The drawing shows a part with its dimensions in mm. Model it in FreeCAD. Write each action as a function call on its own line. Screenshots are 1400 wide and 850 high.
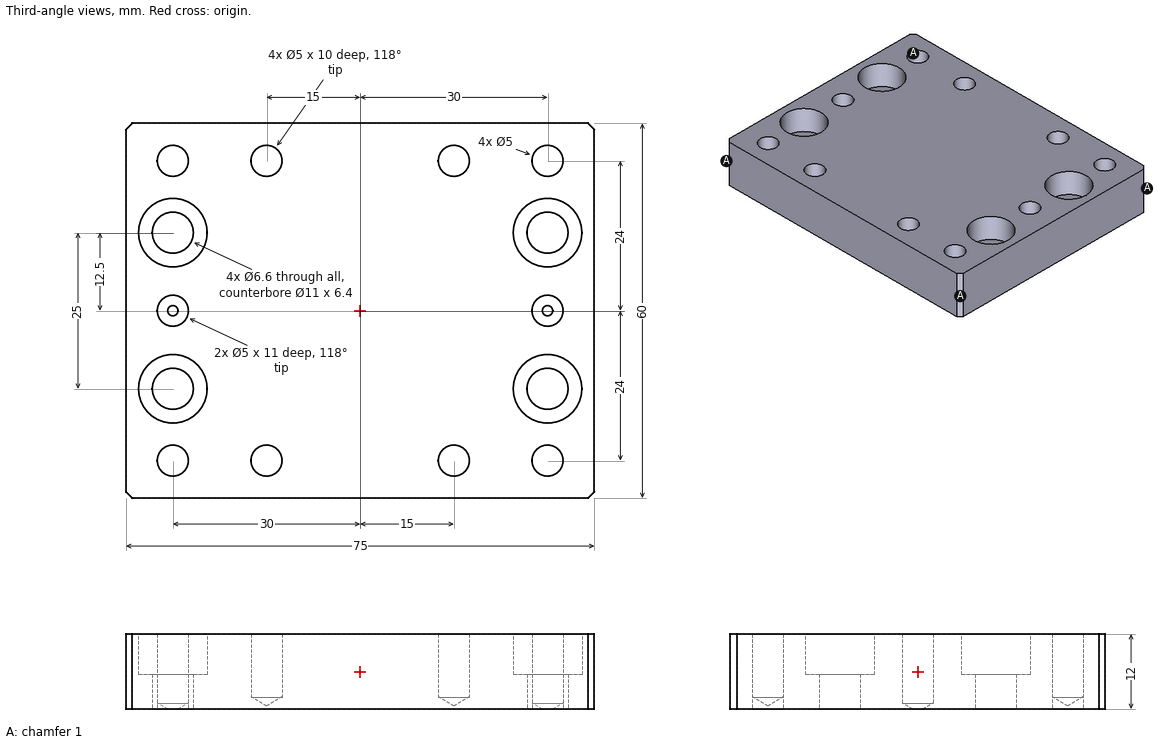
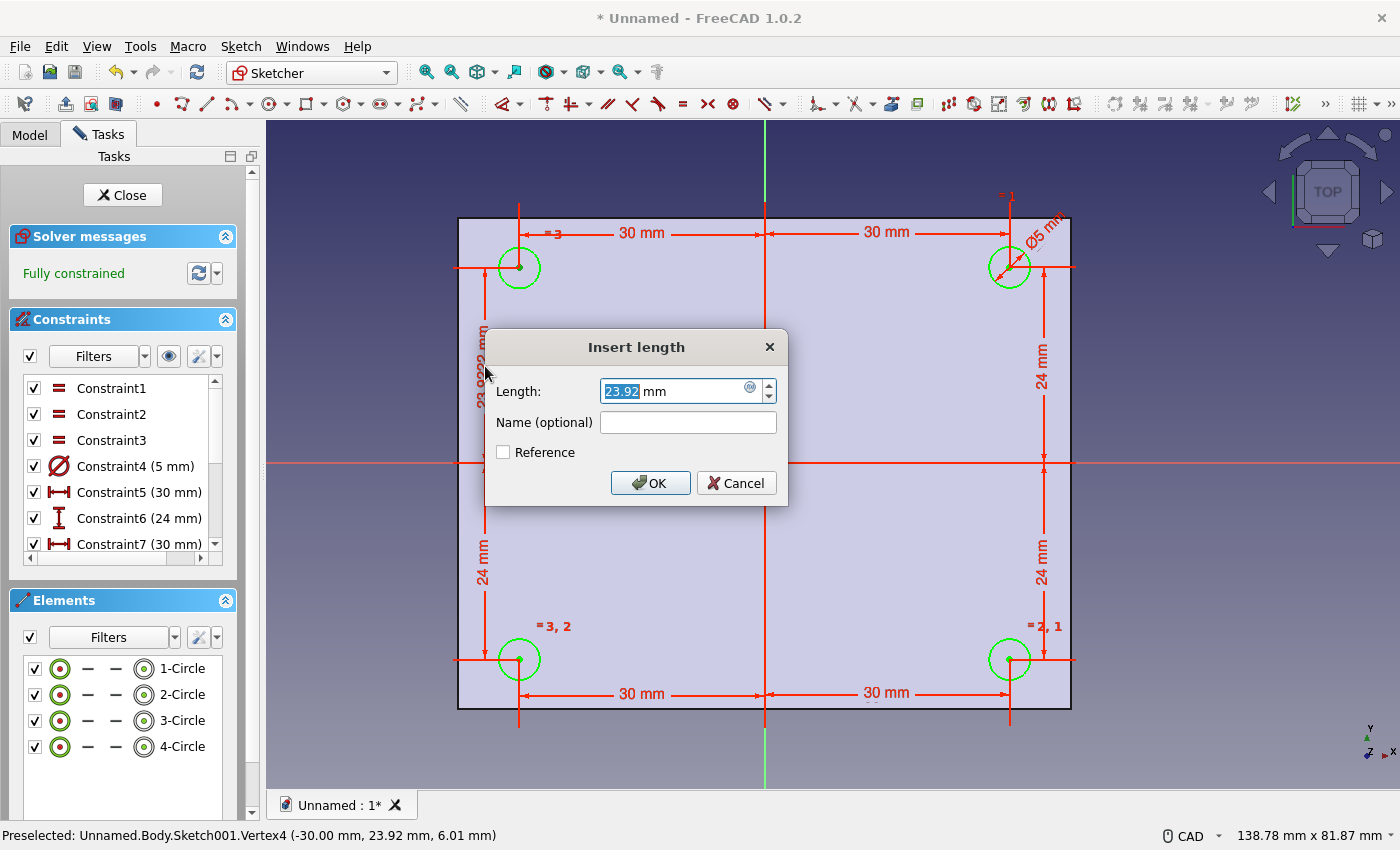
text(24)
key(Return)
key(Escape)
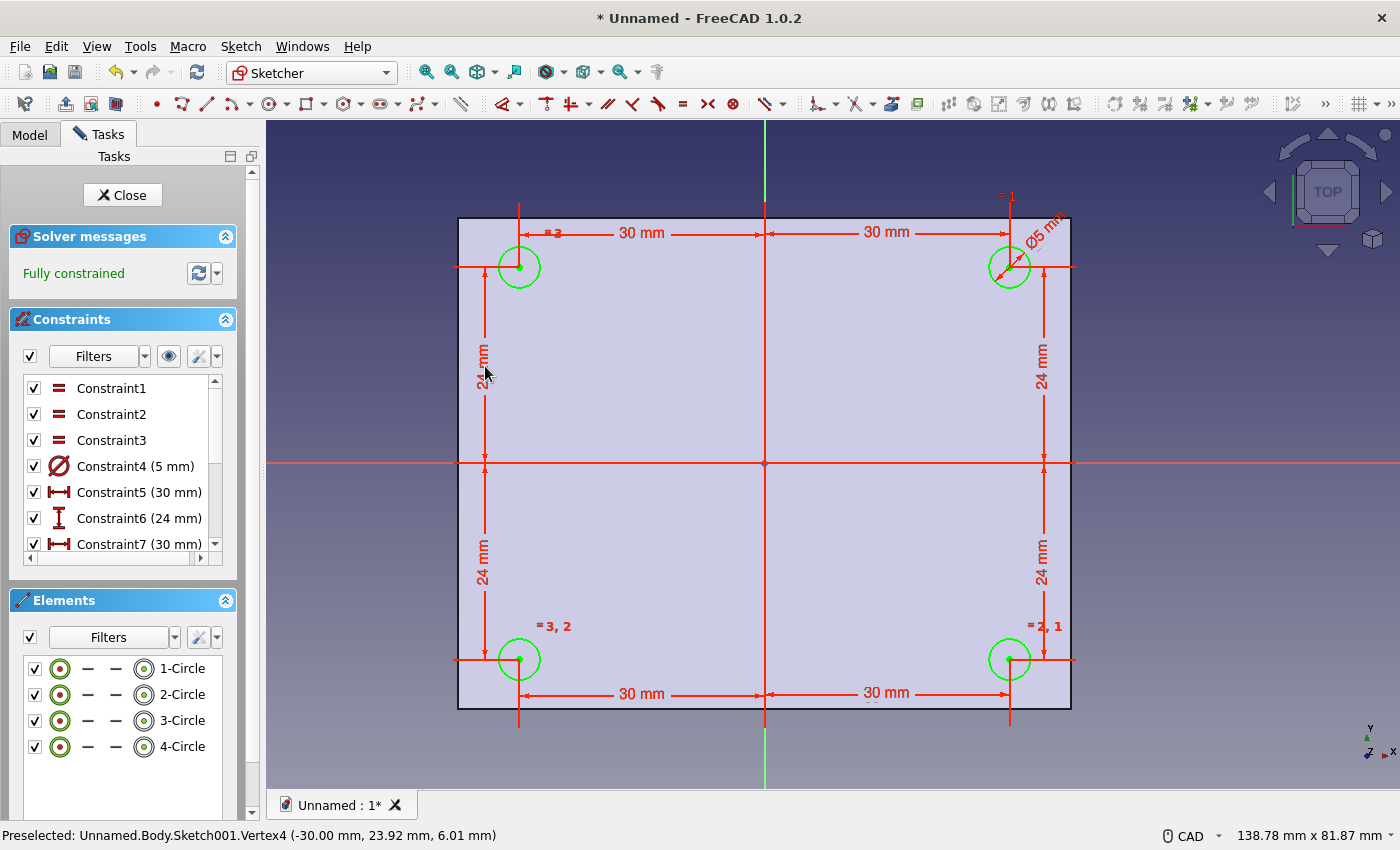
click(123, 195)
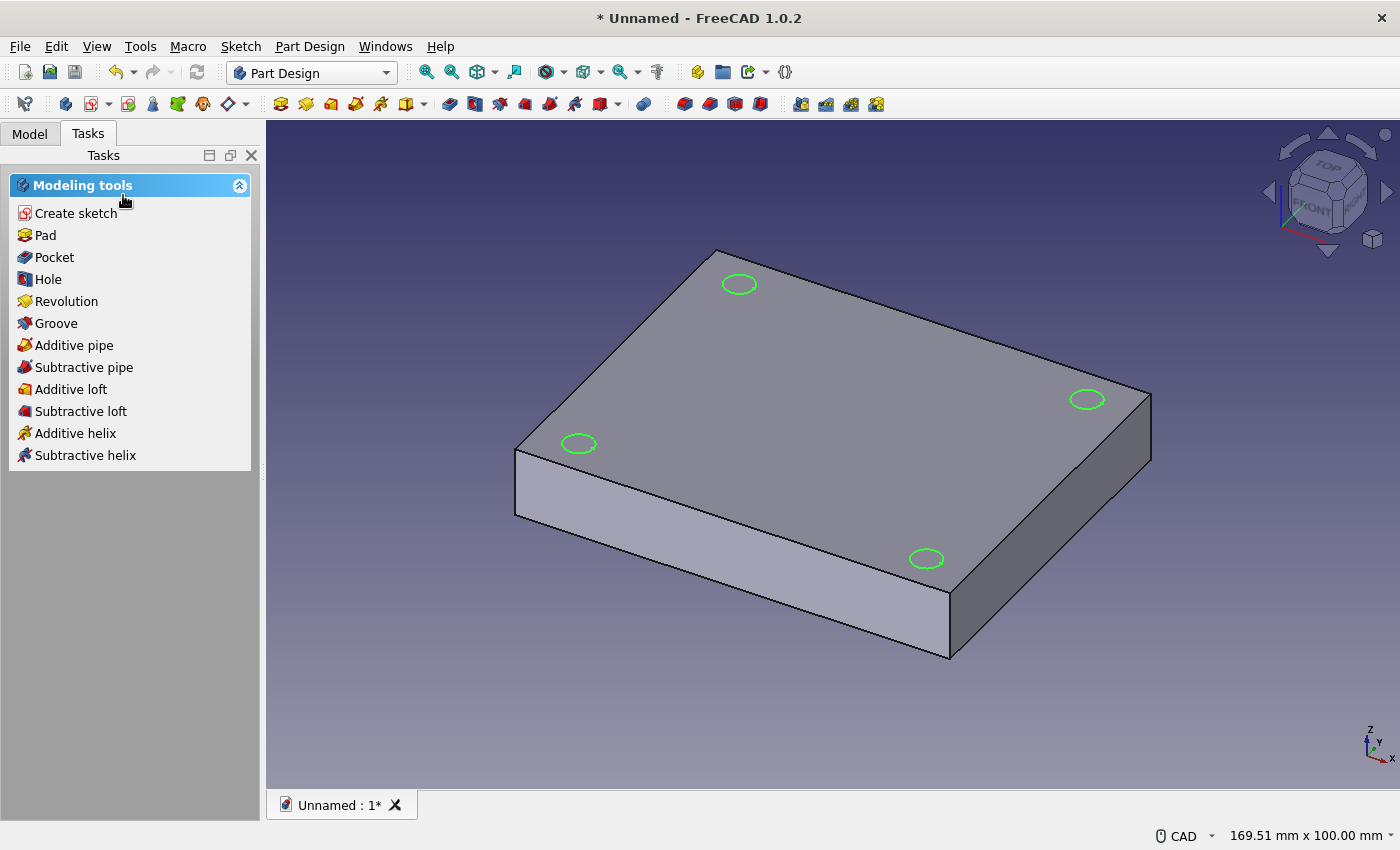
click(450, 104)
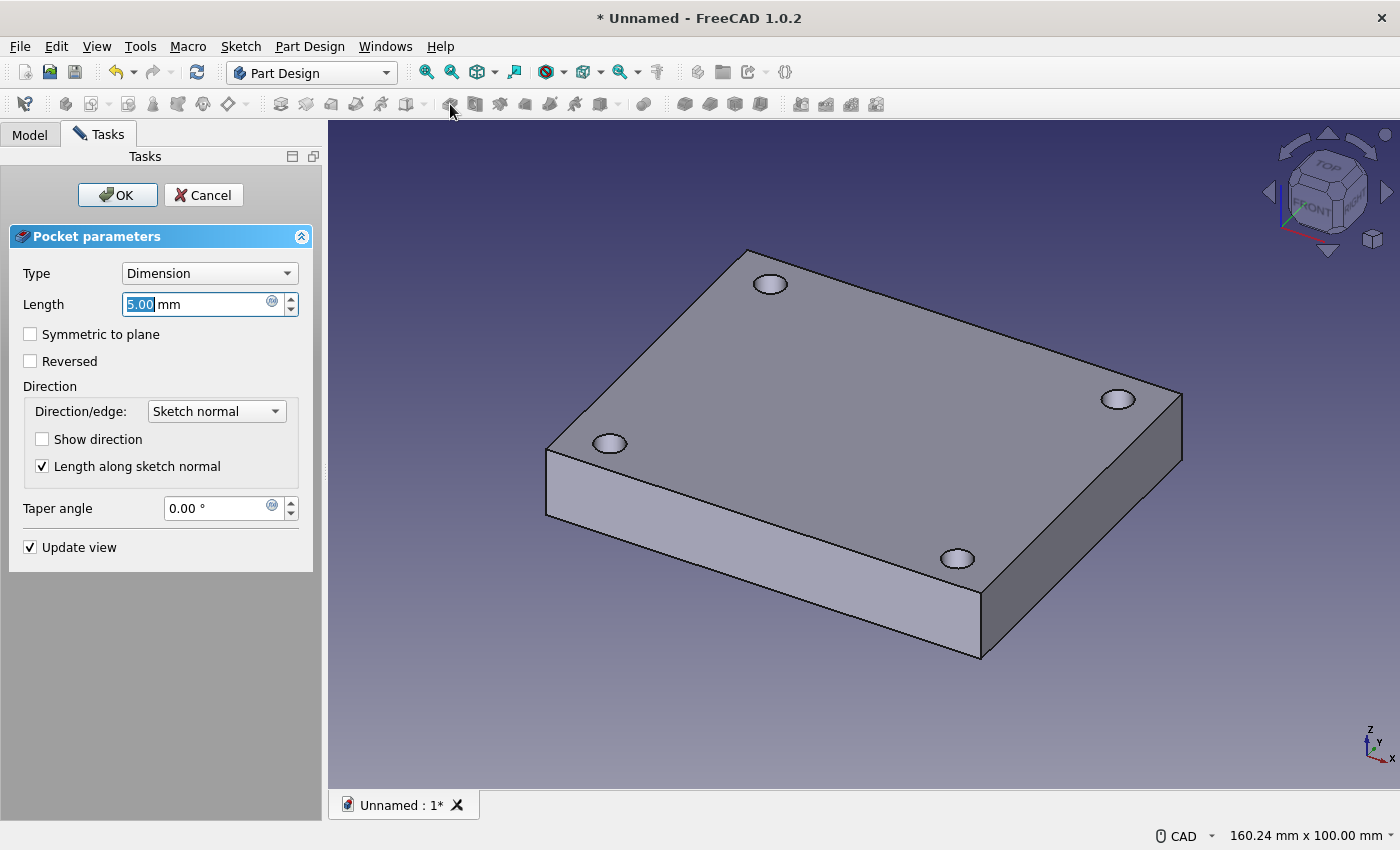
click(210, 274)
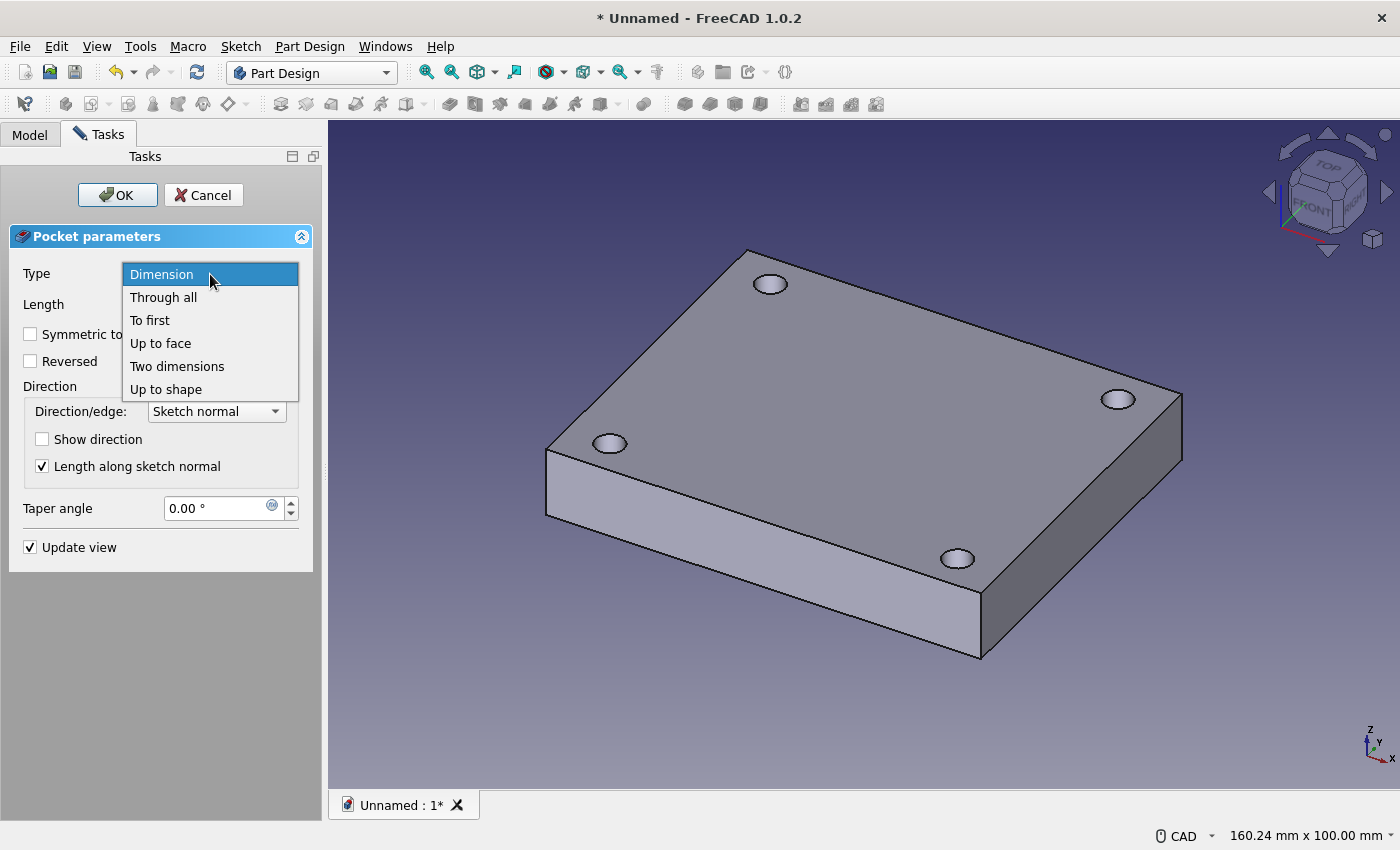
click(208, 298)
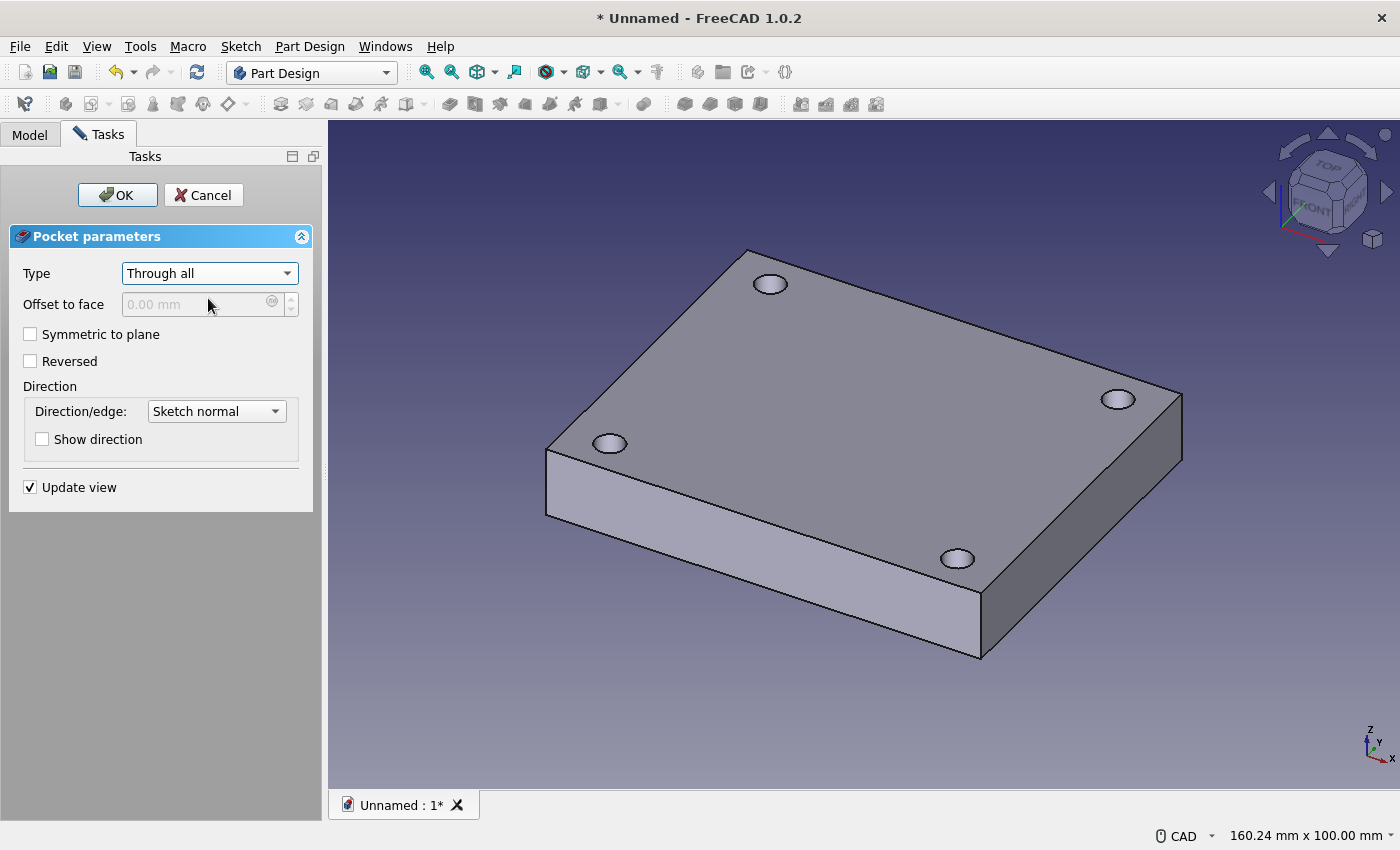
click(118, 195)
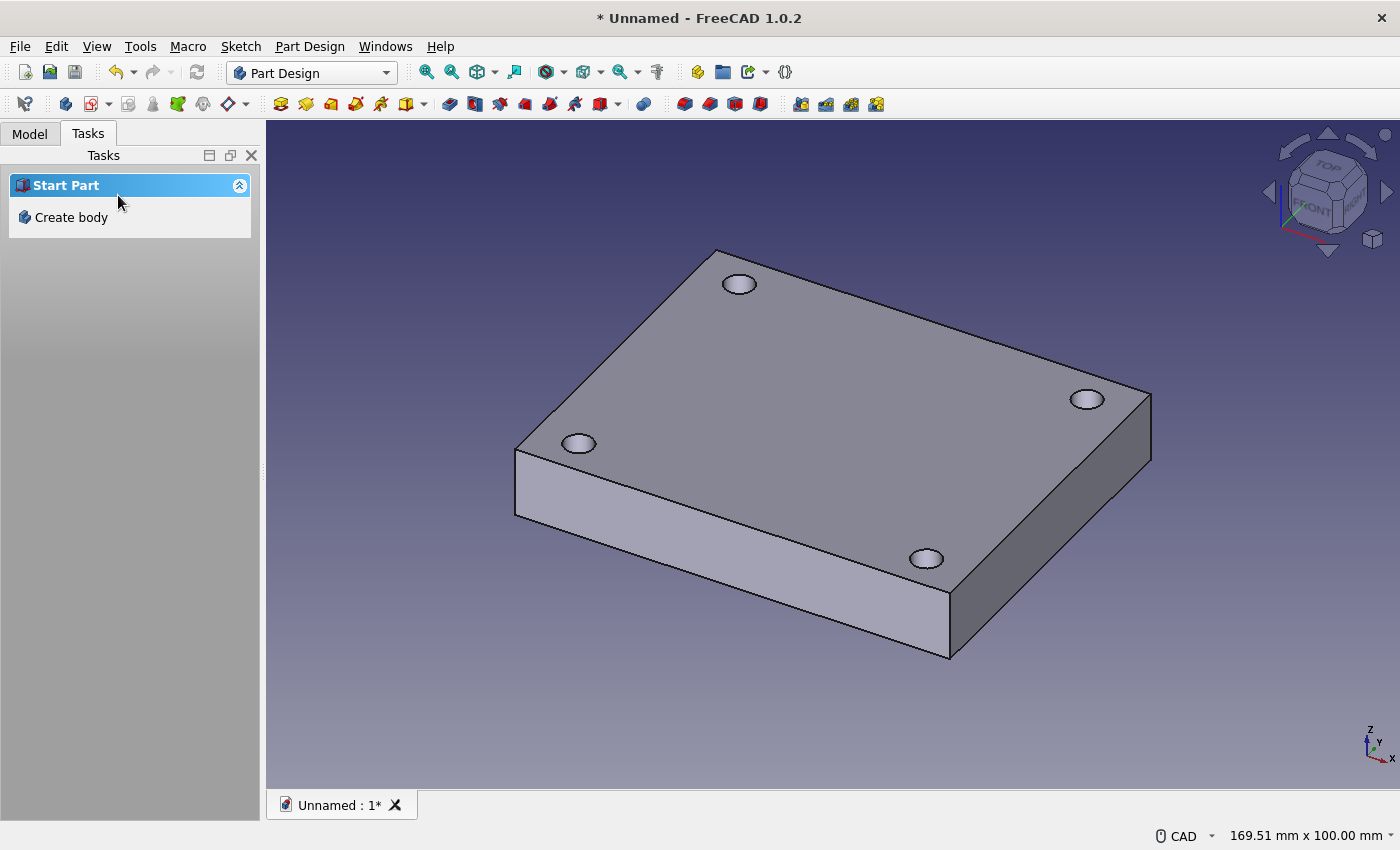
click(833, 421)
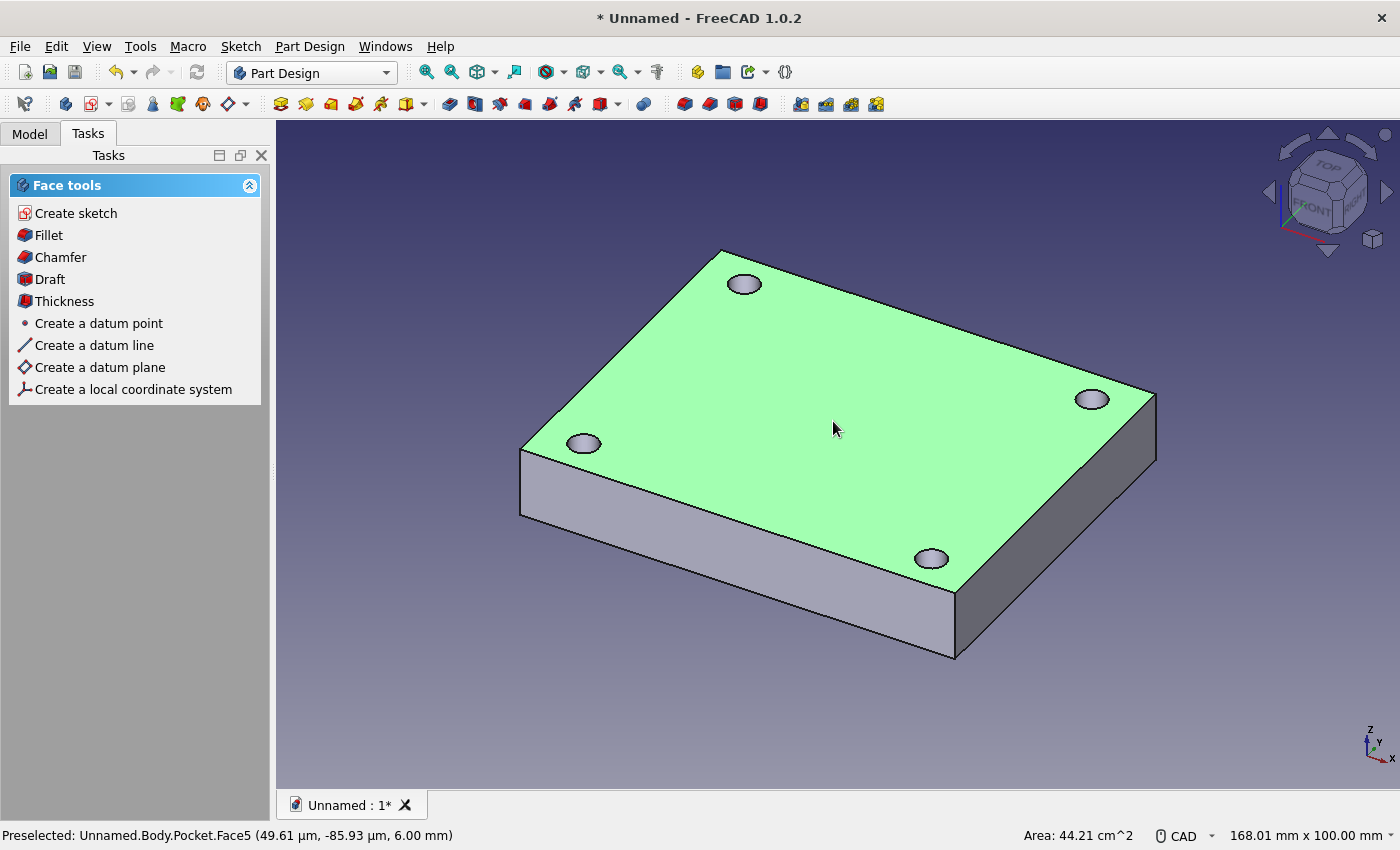
click(90, 104)